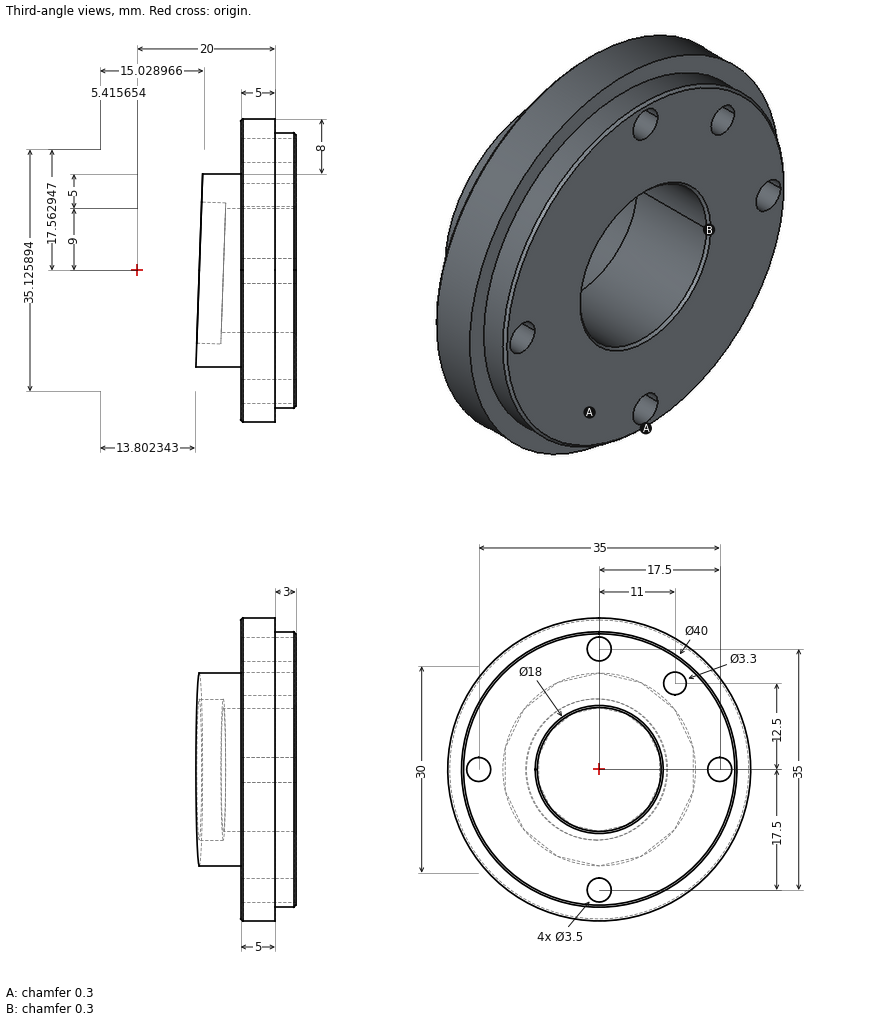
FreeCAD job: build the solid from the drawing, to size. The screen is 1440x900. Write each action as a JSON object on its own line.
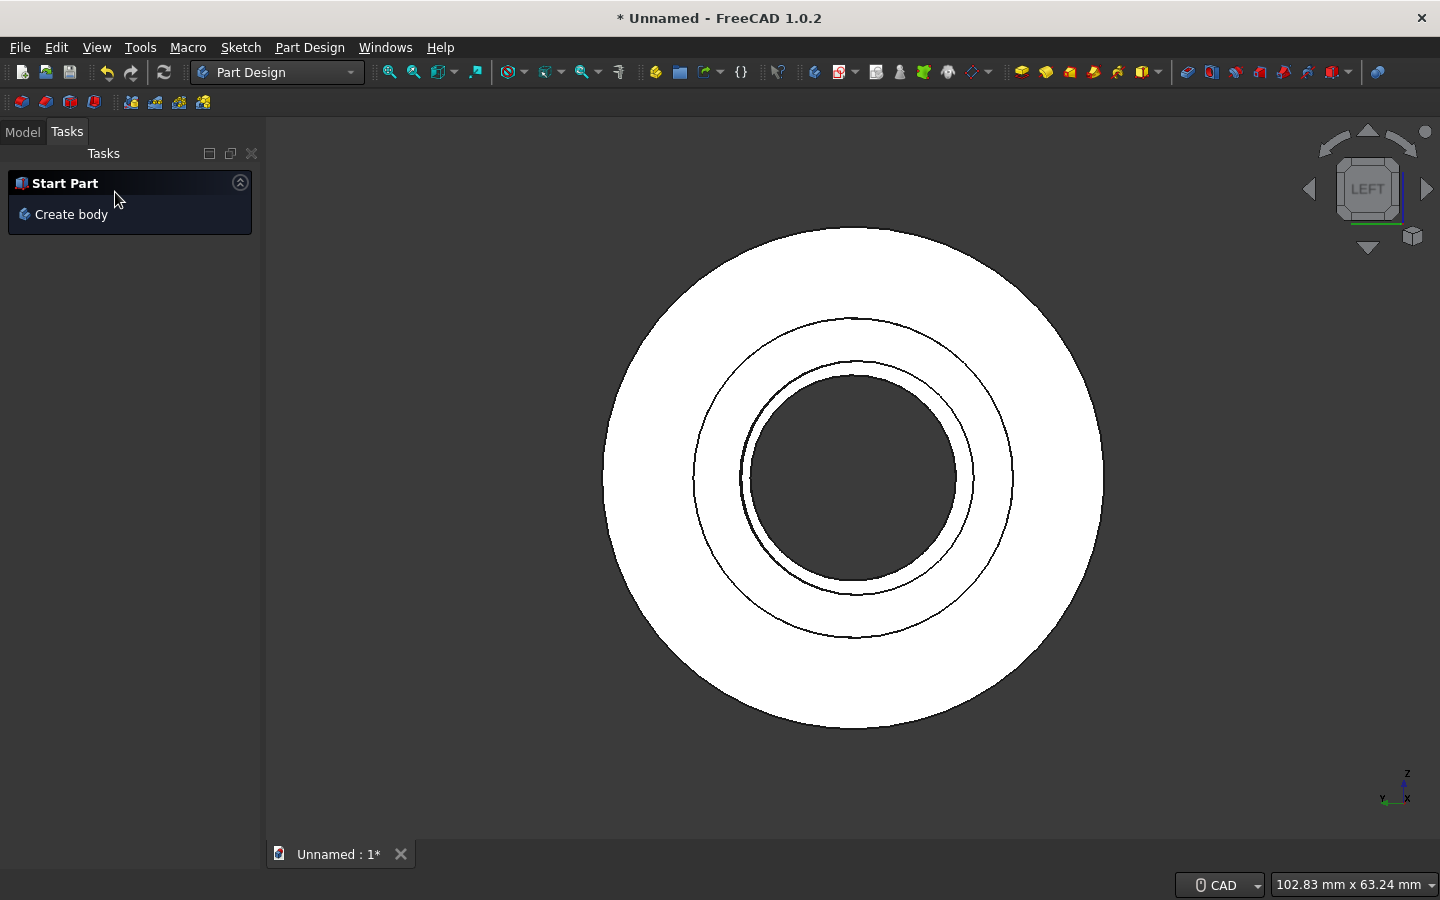
{"action": "left_click", "coordinate": [997, 333]}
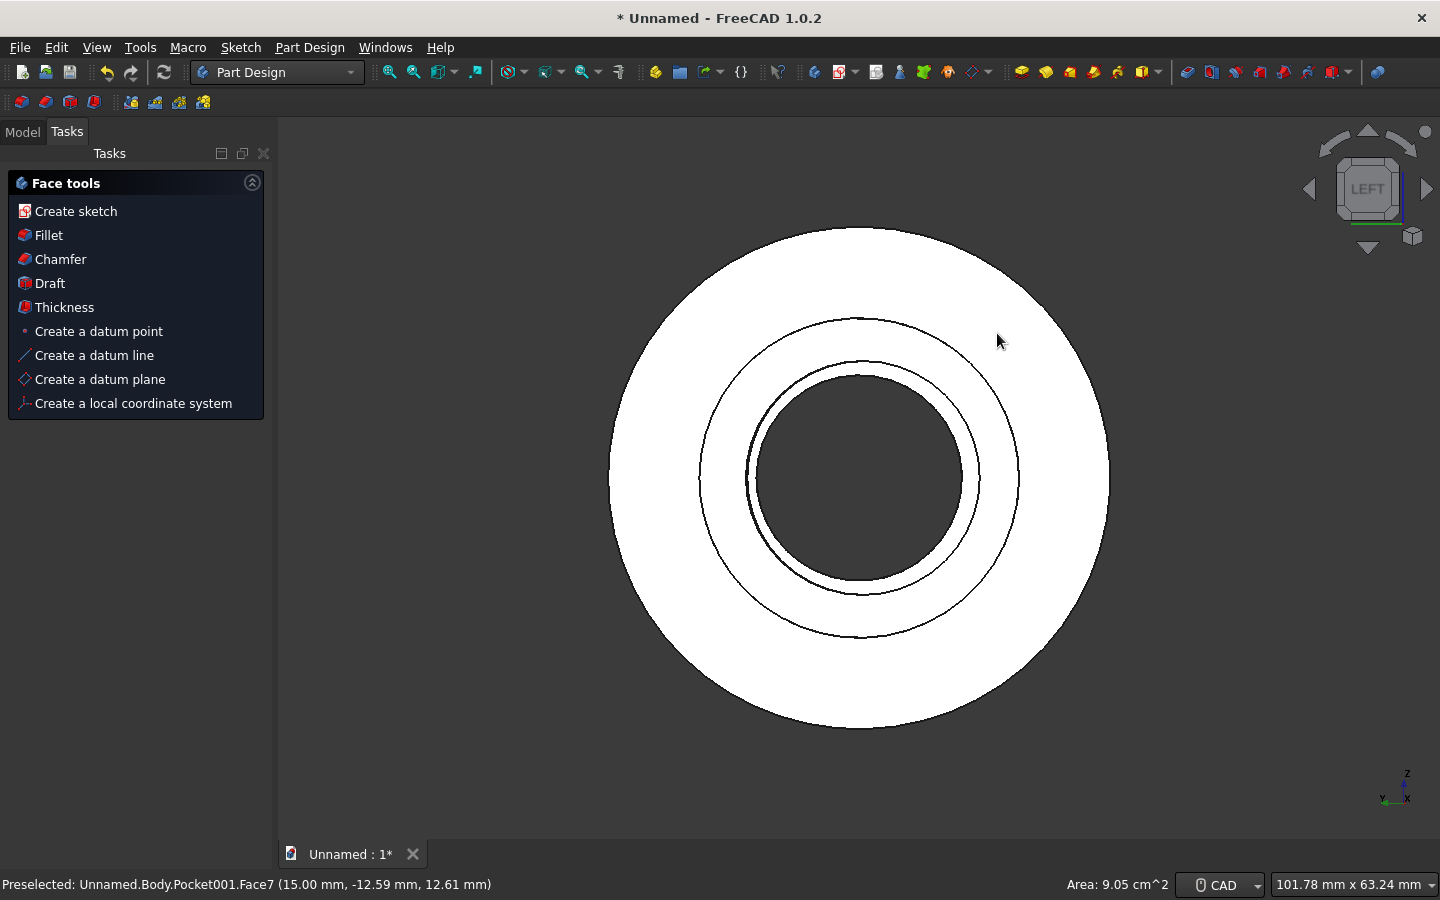
{"action": "left_click", "coordinate": [840, 72]}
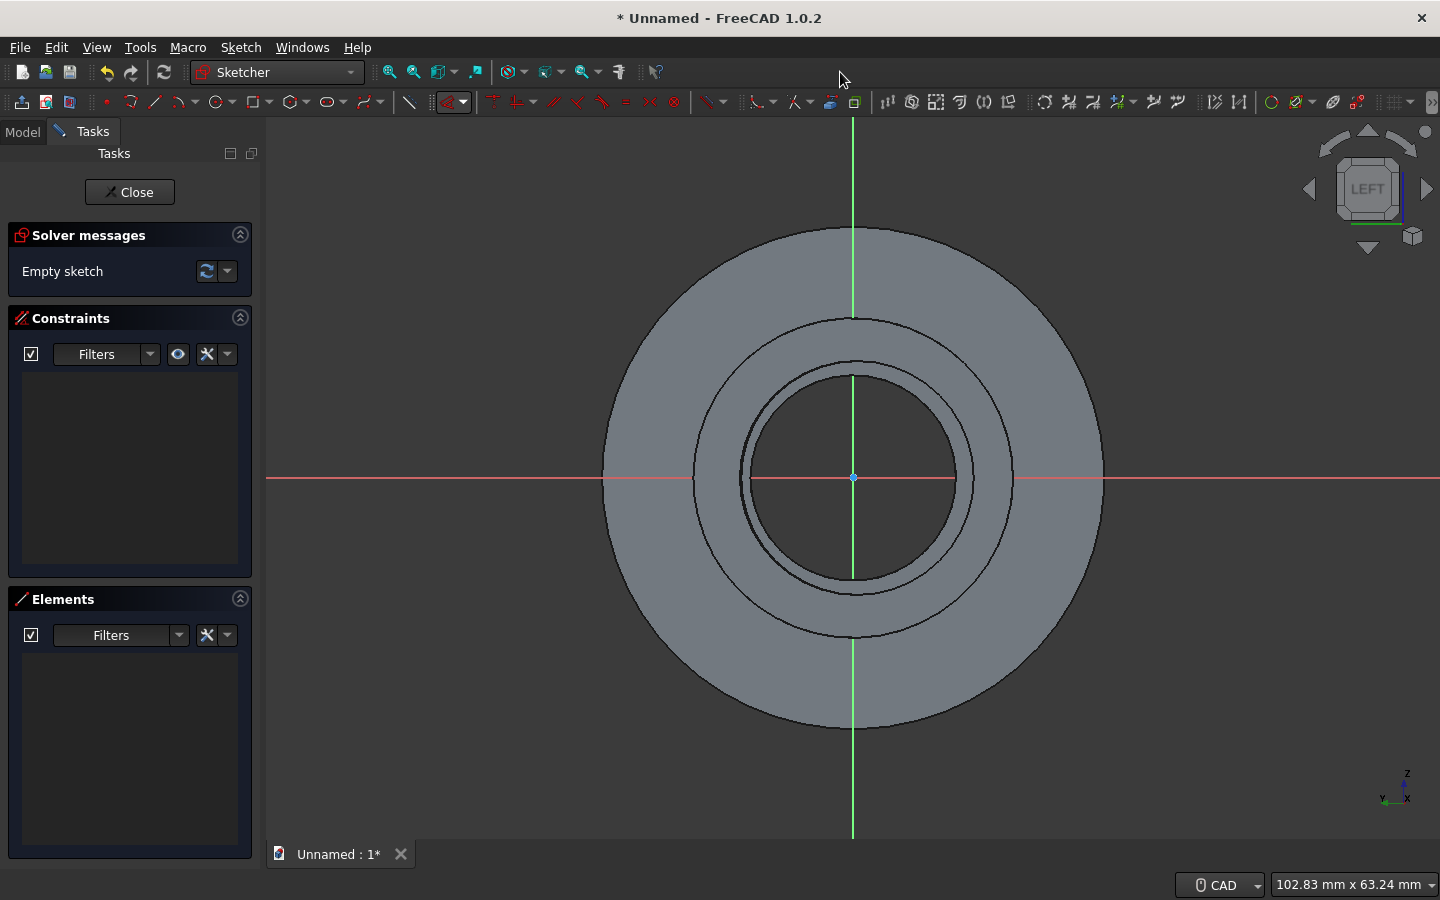
{"action": "key", "text": "g c"}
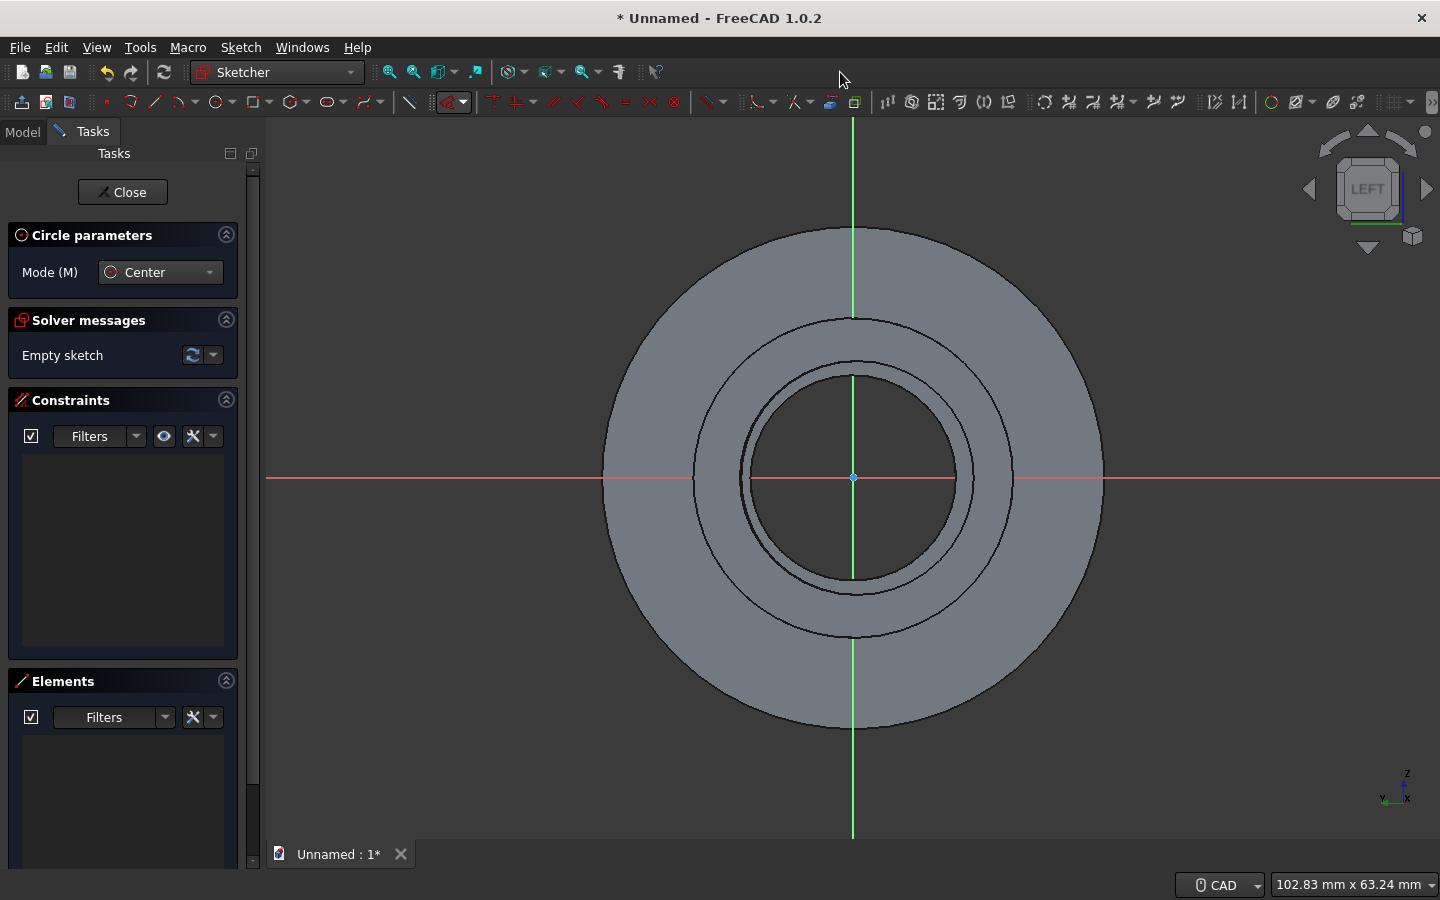
{"action": "left_click", "coordinate": [853, 678]}
{"action": "mouse_move", "coordinate": [867, 664]}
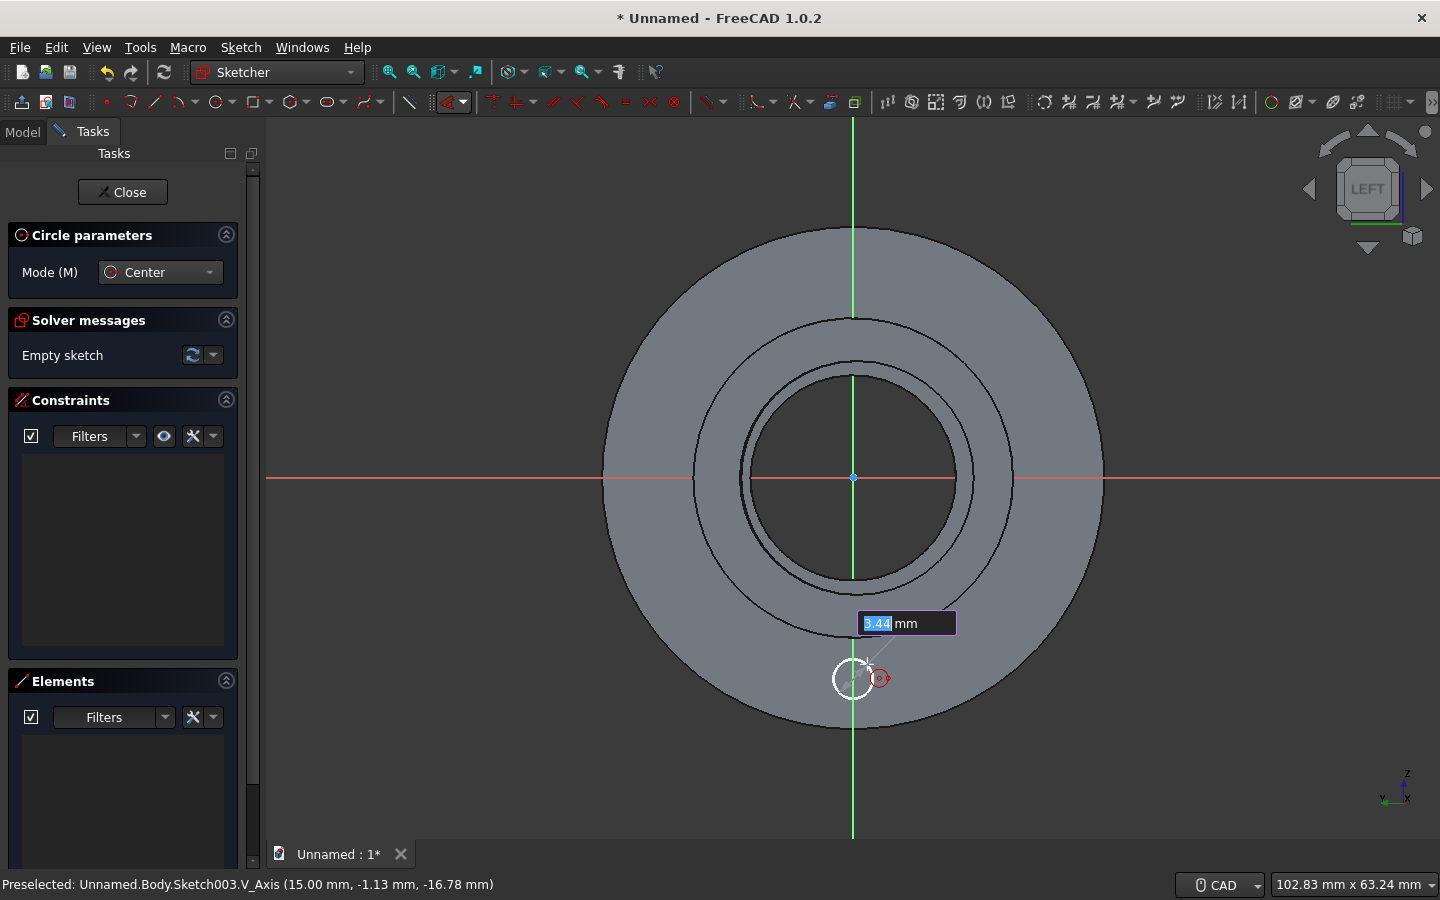
{"action": "type", "text": "3.5"}
{"action": "key", "text": "Return"}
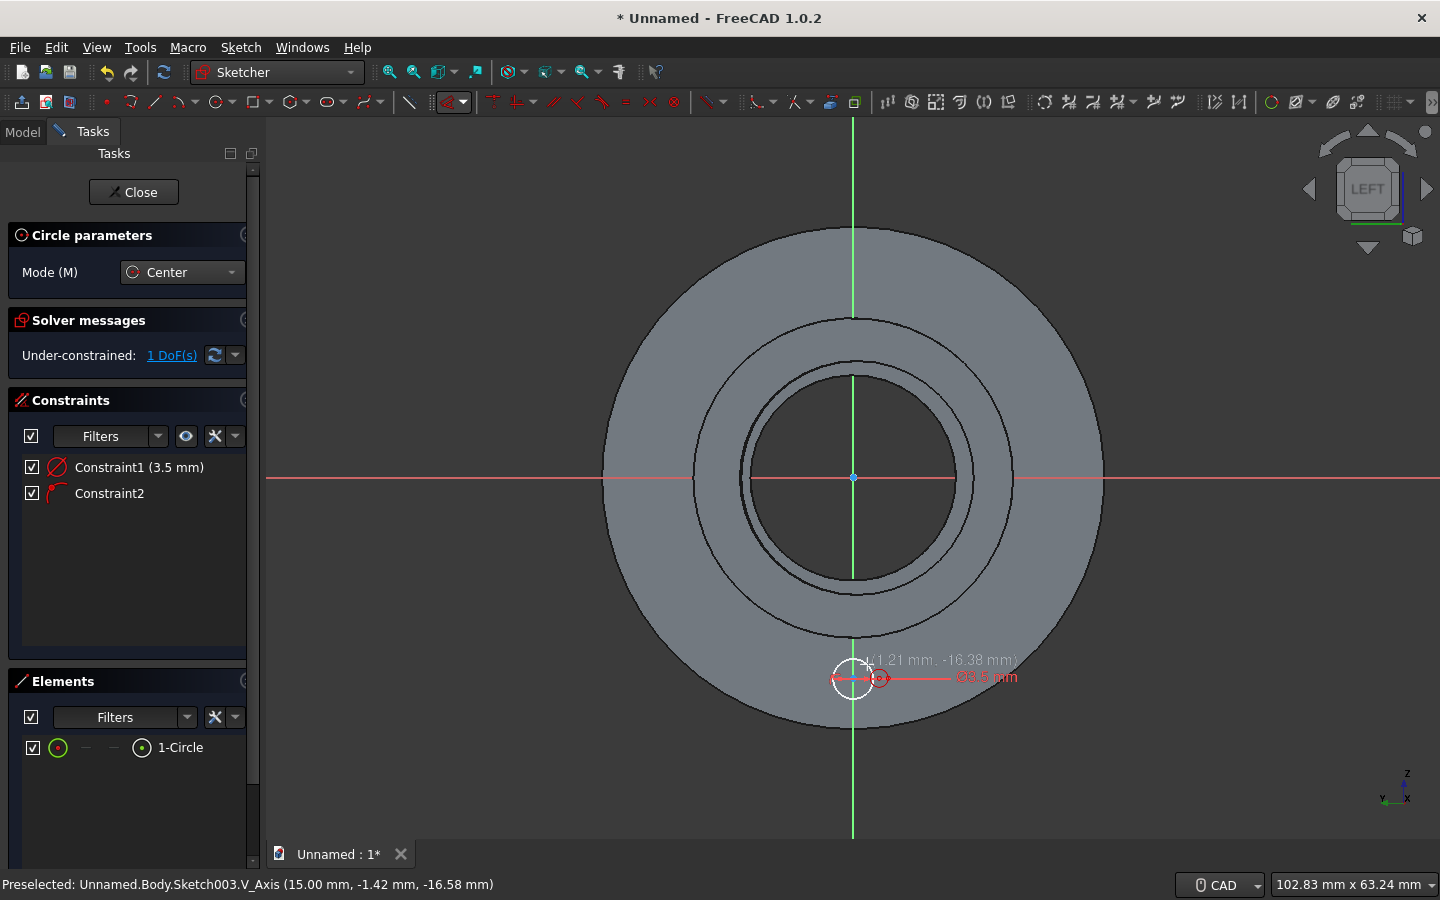
{"action": "left_click", "coordinate": [653, 478]}
{"action": "mouse_move", "coordinate": [668, 464]}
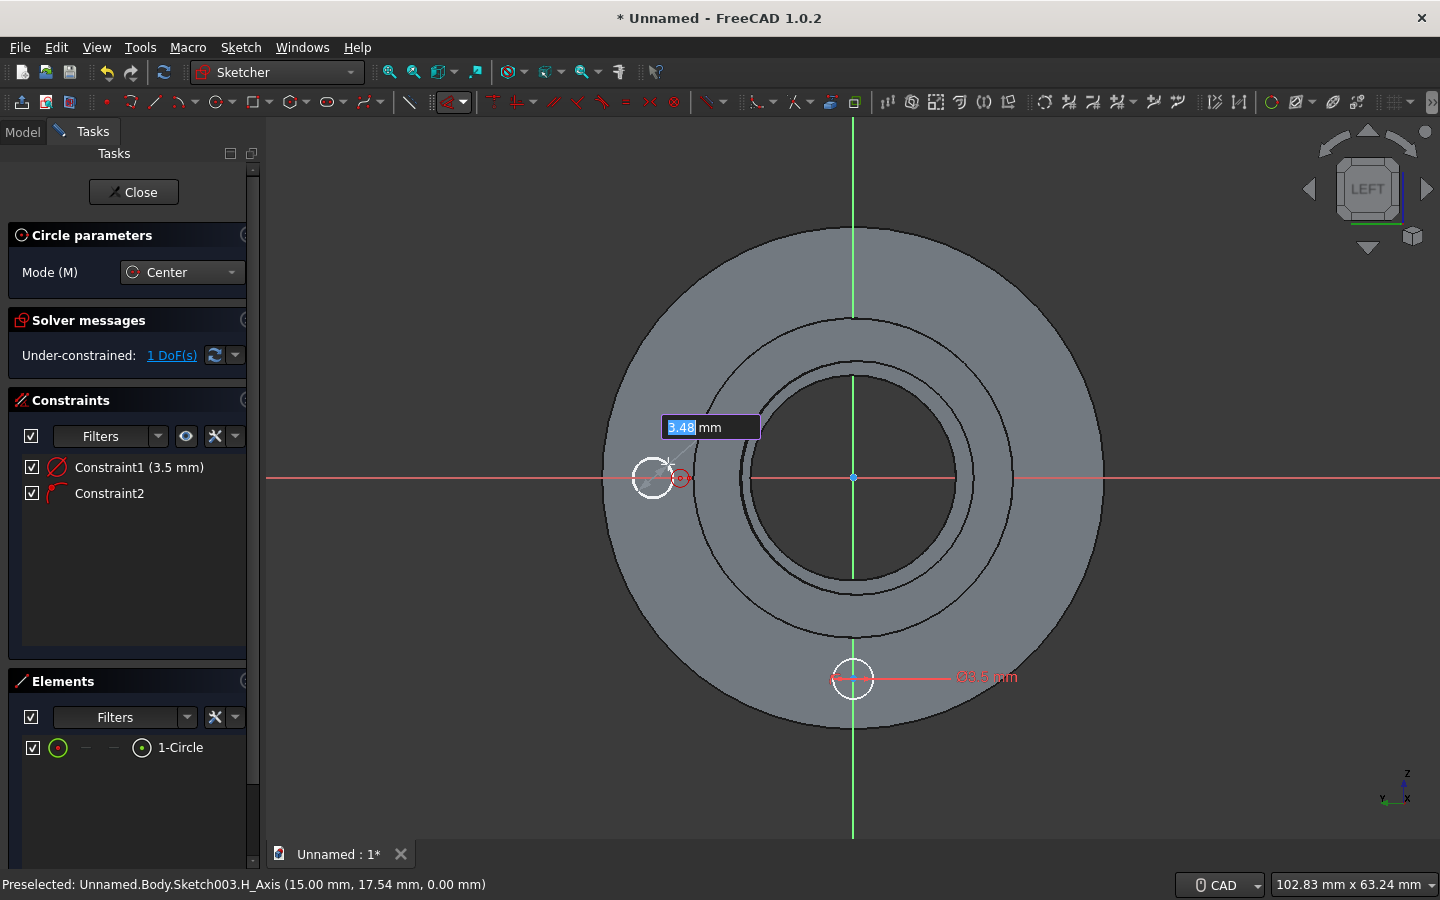
{"action": "type", "text": "3.5"}
{"action": "key", "text": "Return"}